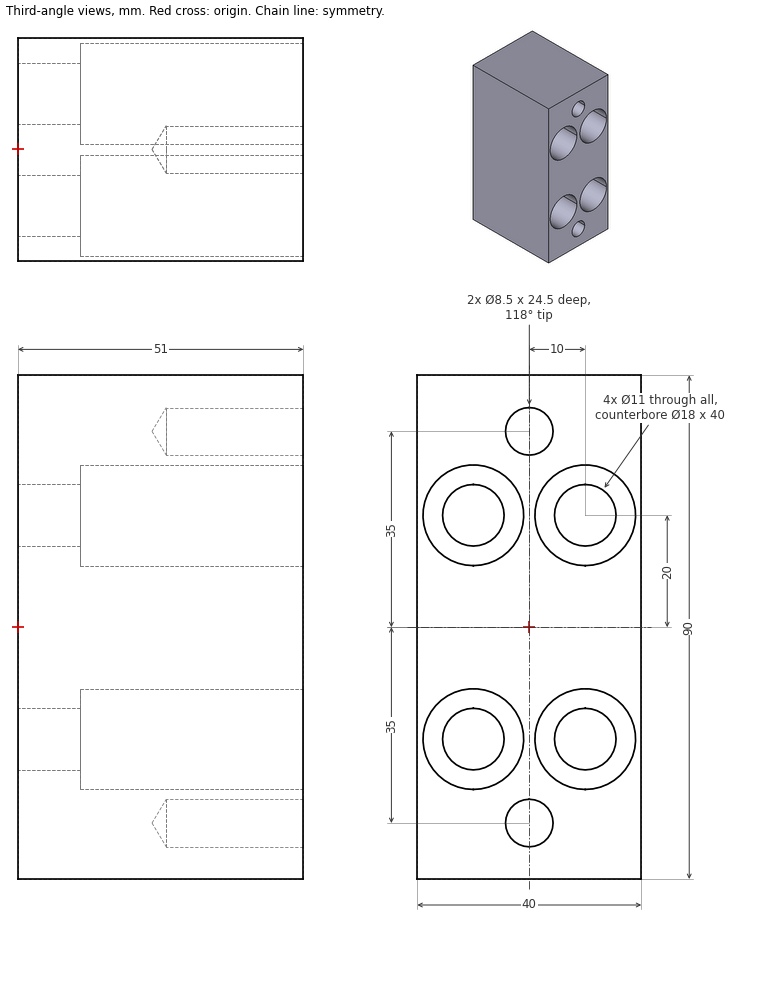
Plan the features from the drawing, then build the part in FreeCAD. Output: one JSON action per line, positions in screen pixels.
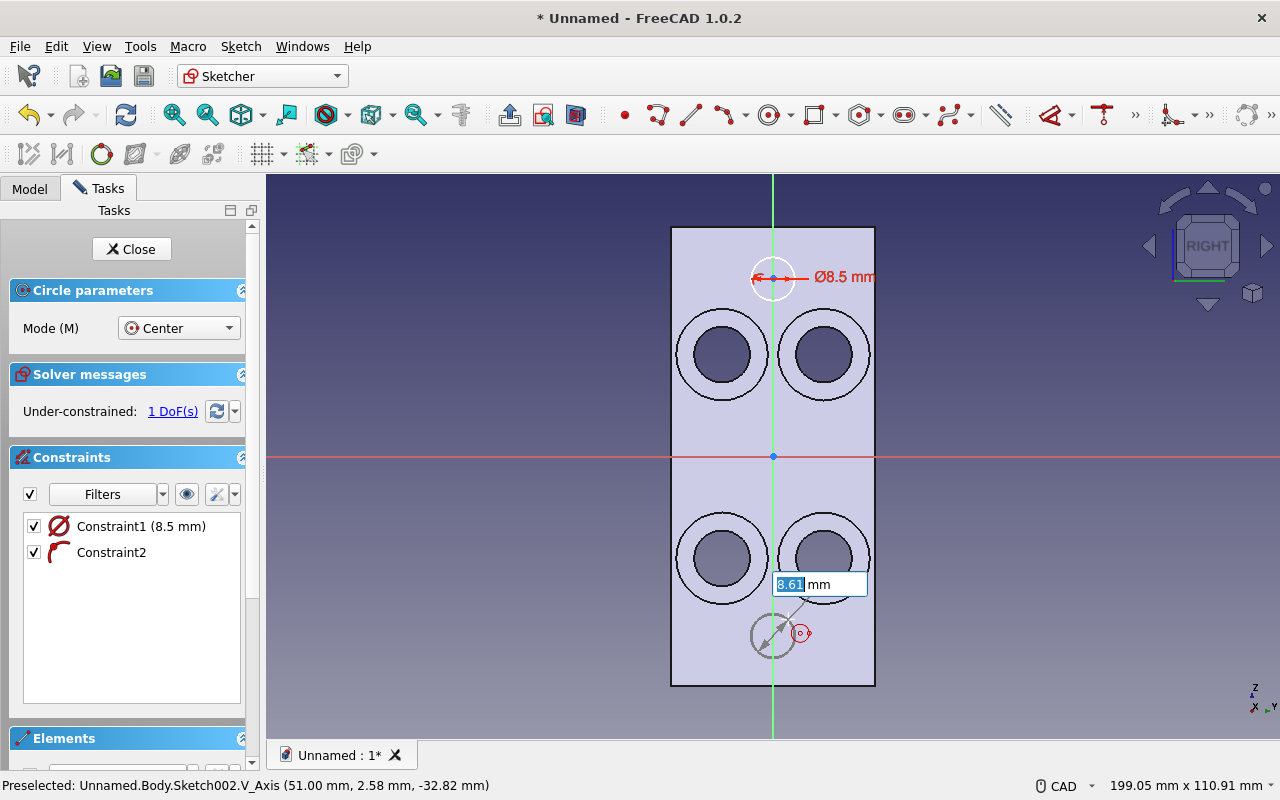
{"action": "type", "text": "8.5"}
{"action": "key", "text": "Return"}
{"action": "key", "text": "Escape"}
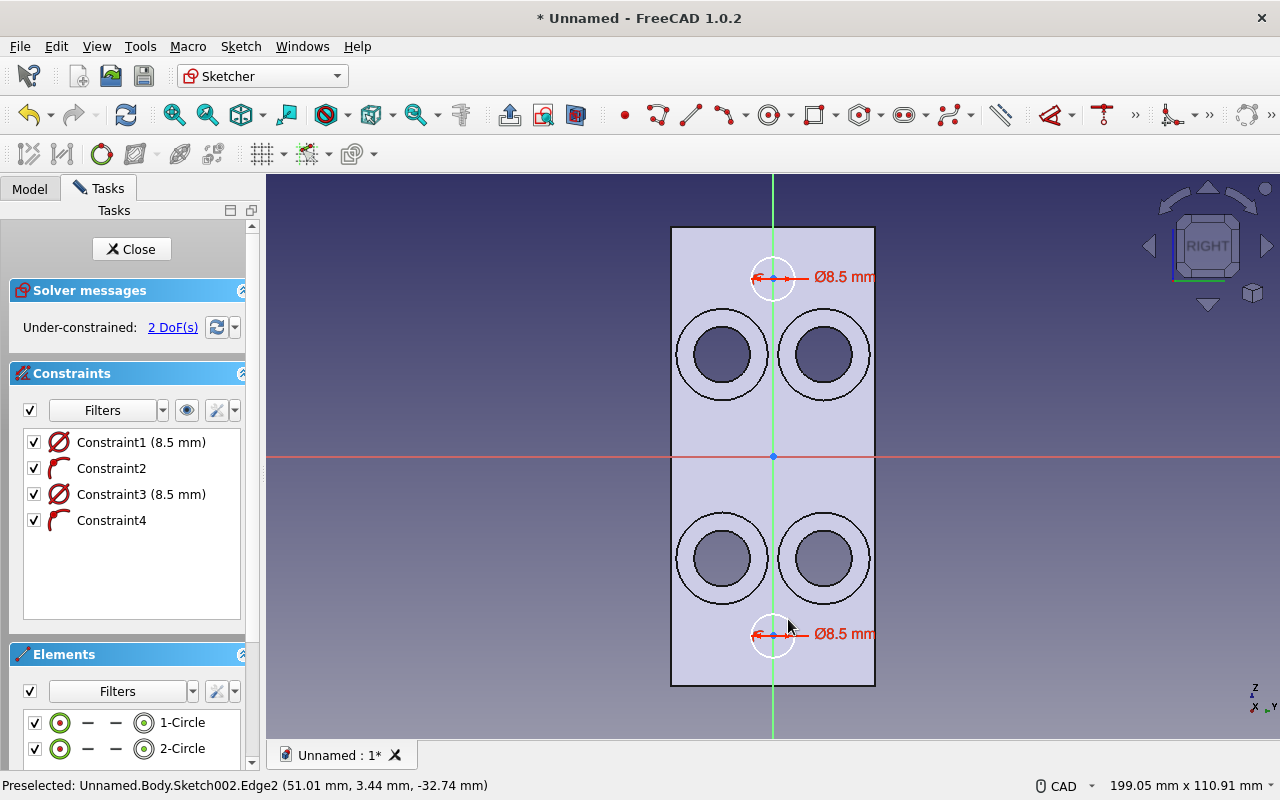
{"action": "key", "text": "d"}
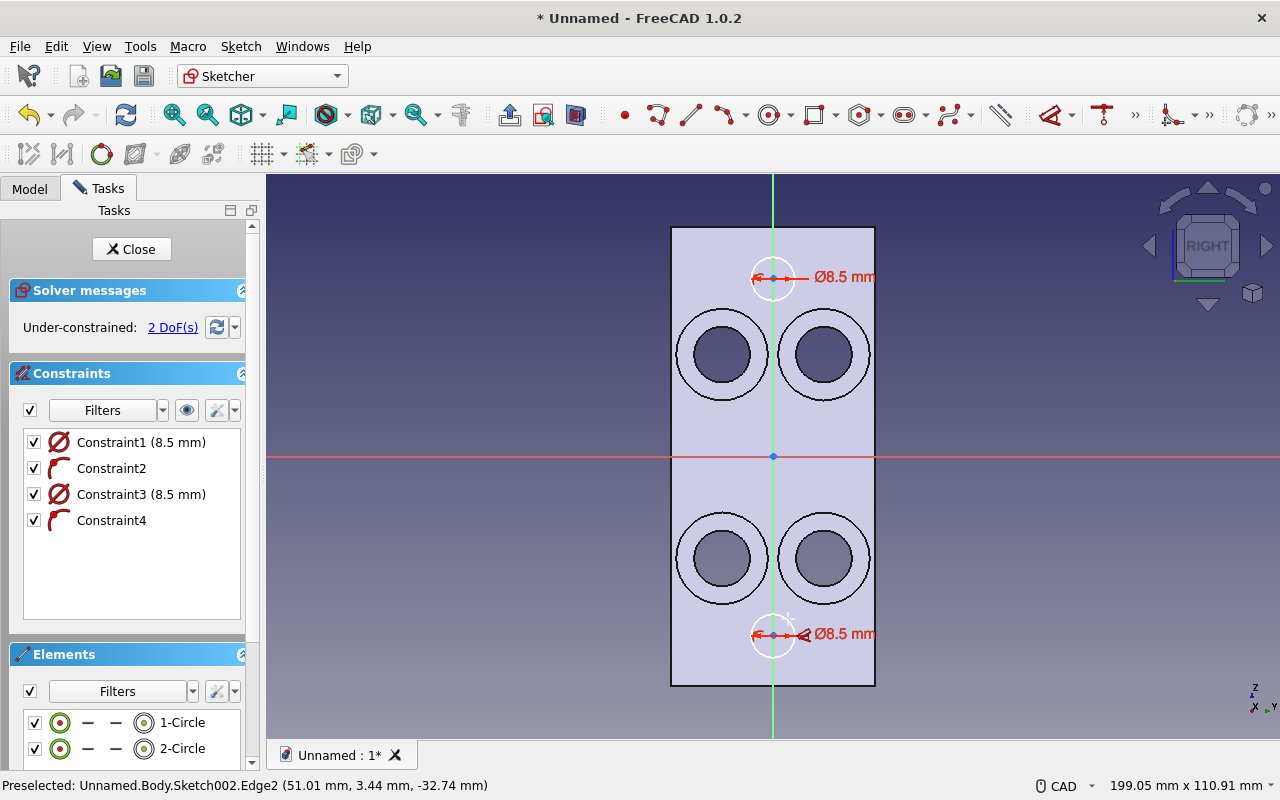
{"action": "left_click", "coordinate": [773, 279]}
{"action": "left_click", "coordinate": [807, 368]}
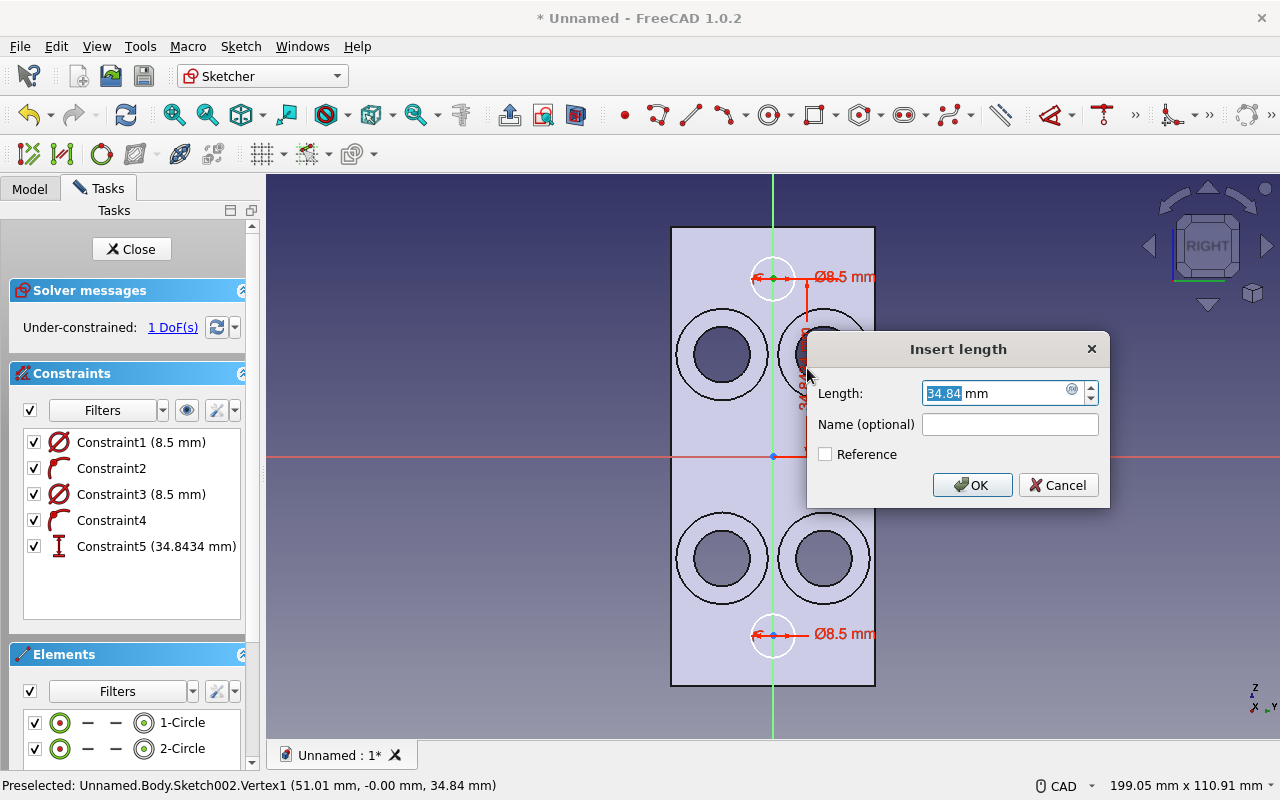
{"action": "type", "text": "35"}
{"action": "key", "text": "Return"}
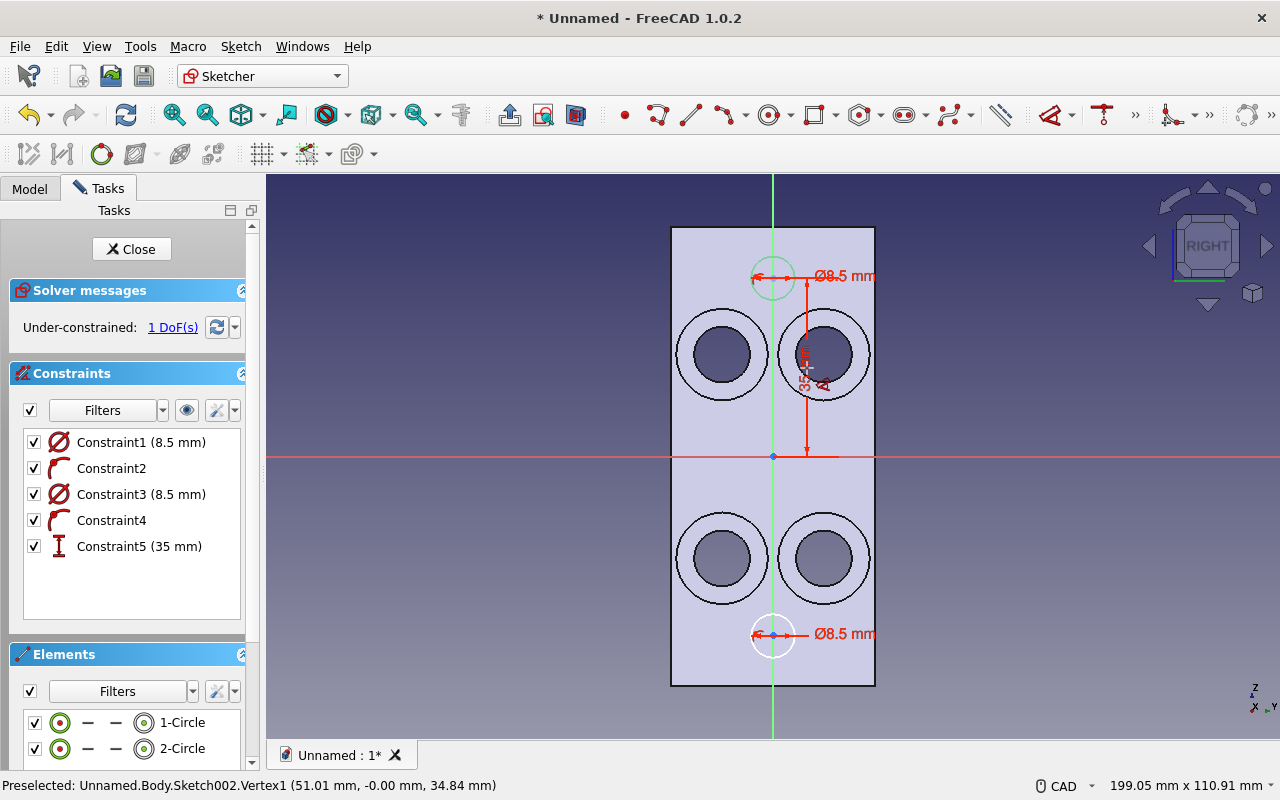
{"action": "left_click", "coordinate": [773, 636]}
{"action": "left_click", "coordinate": [807, 546]}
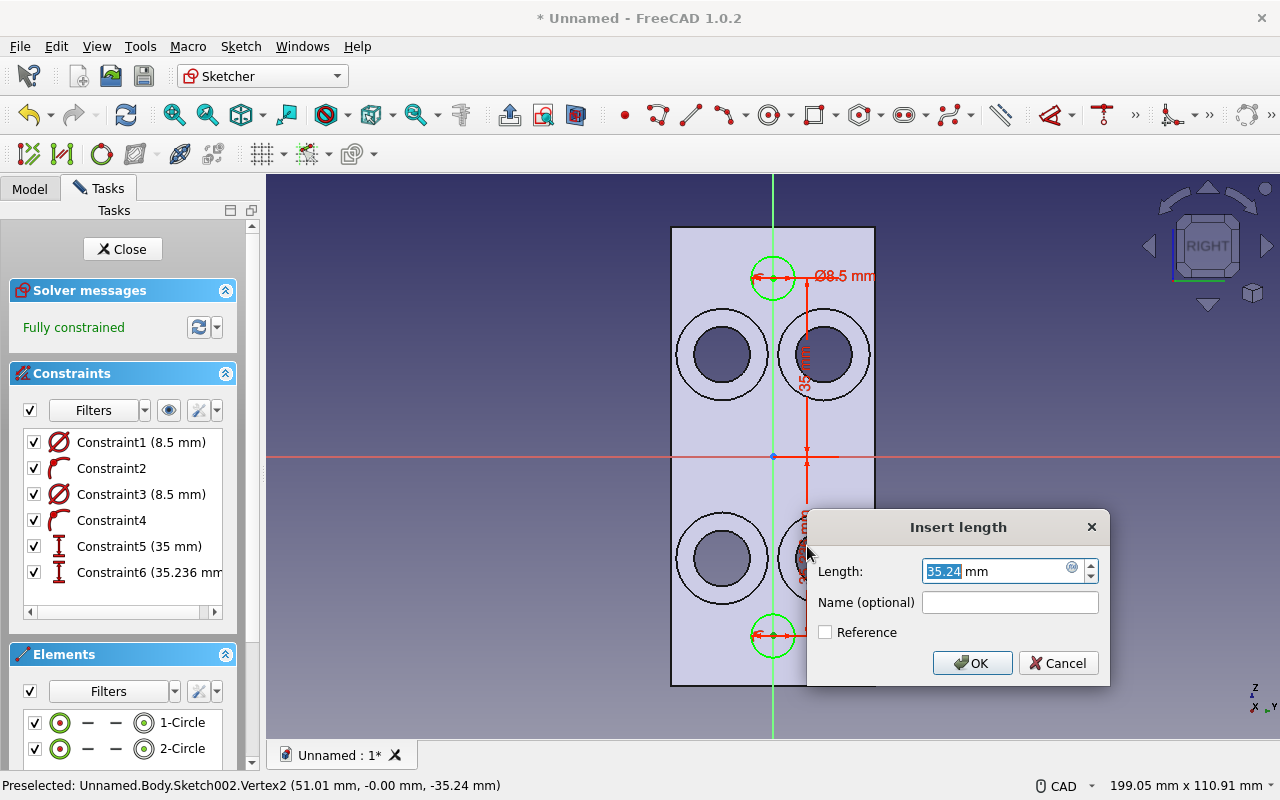
{"action": "type", "text": "35"}
{"action": "key", "text": "Return"}
{"action": "key", "text": "Escape"}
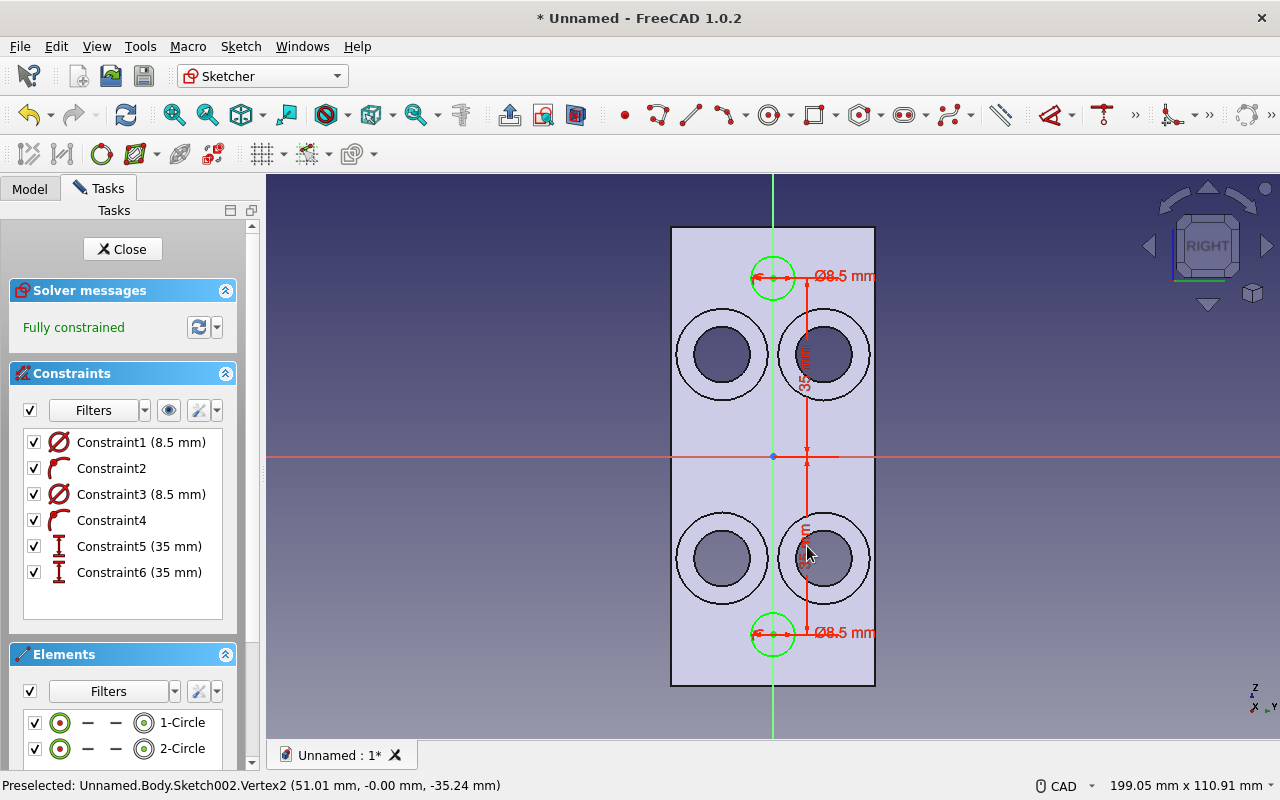
{"action": "left_click", "coordinate": [123, 249]}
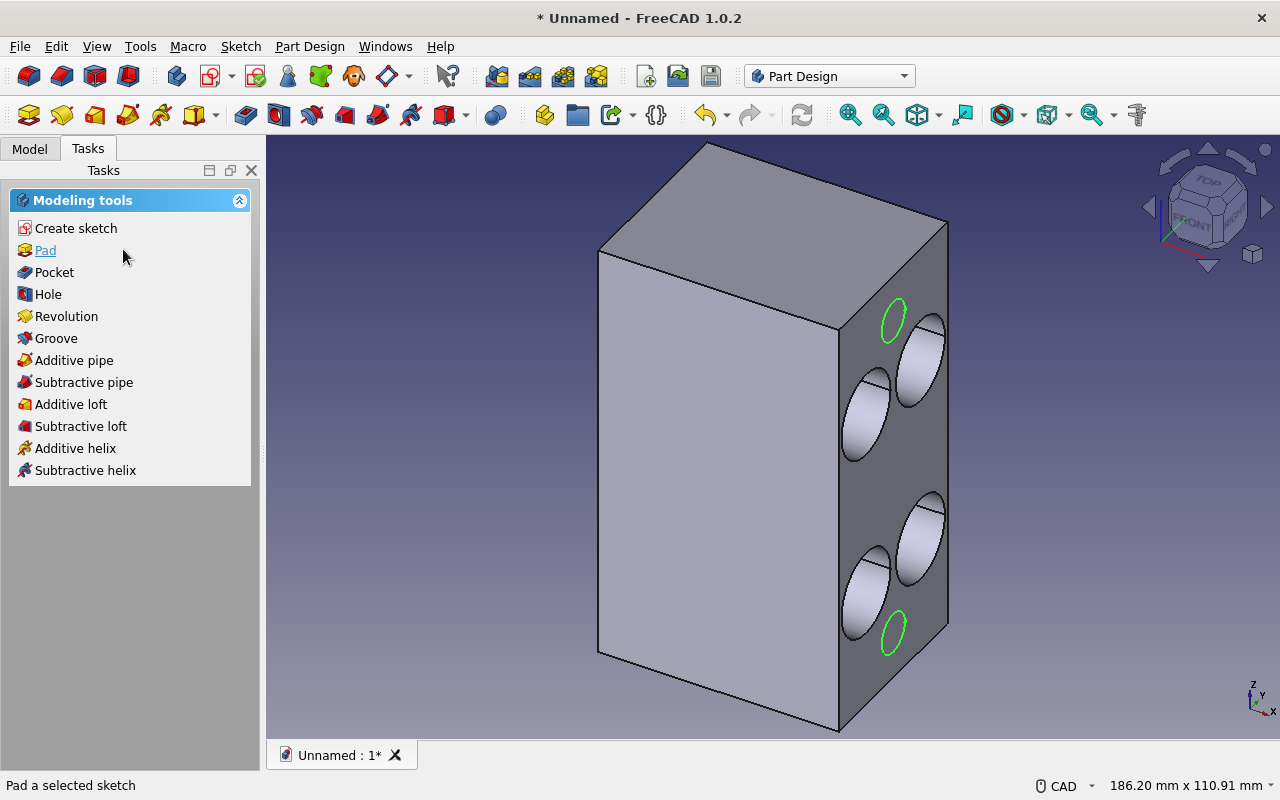
{"action": "left_click", "coordinate": [279, 116]}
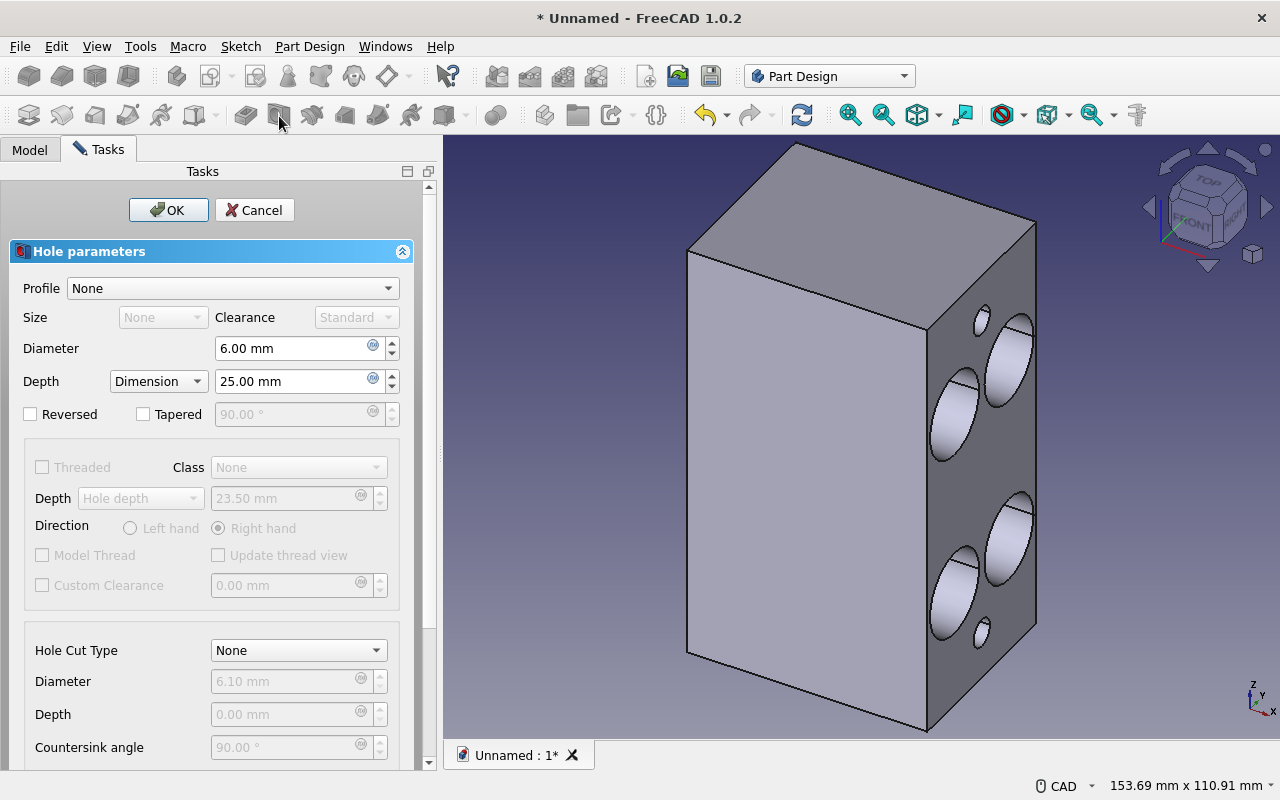
{"action": "triple_click", "coordinate": [300, 348]}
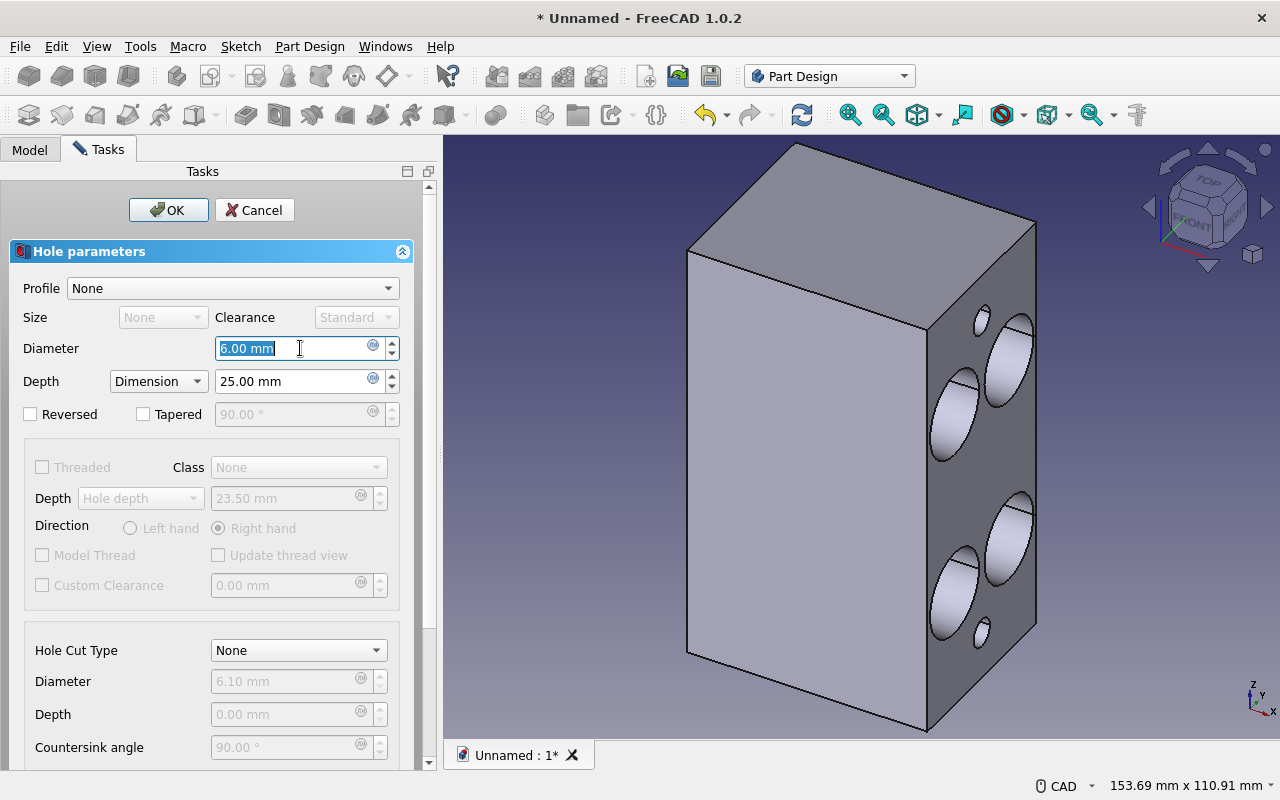
{"action": "type", "text": "8.5"}
{"action": "key", "text": "Tab"}